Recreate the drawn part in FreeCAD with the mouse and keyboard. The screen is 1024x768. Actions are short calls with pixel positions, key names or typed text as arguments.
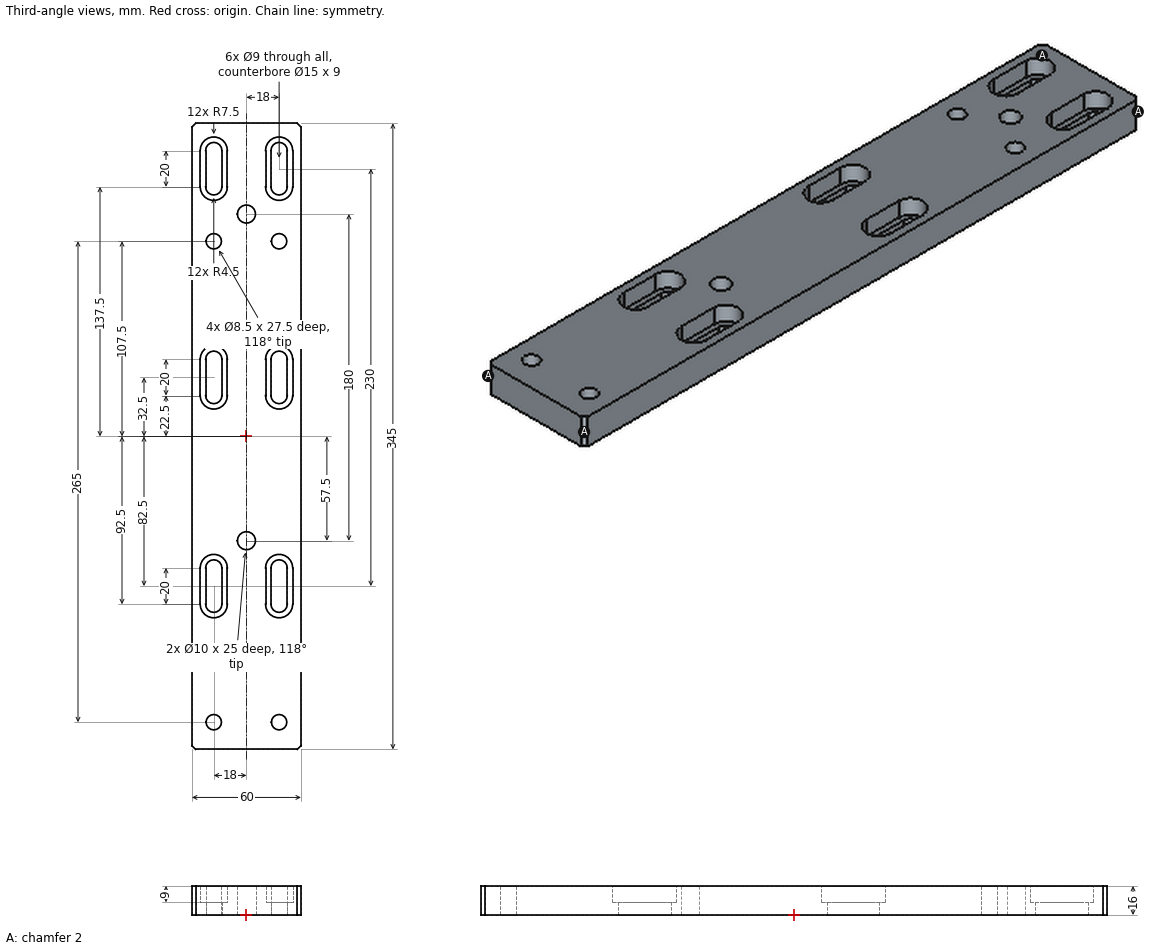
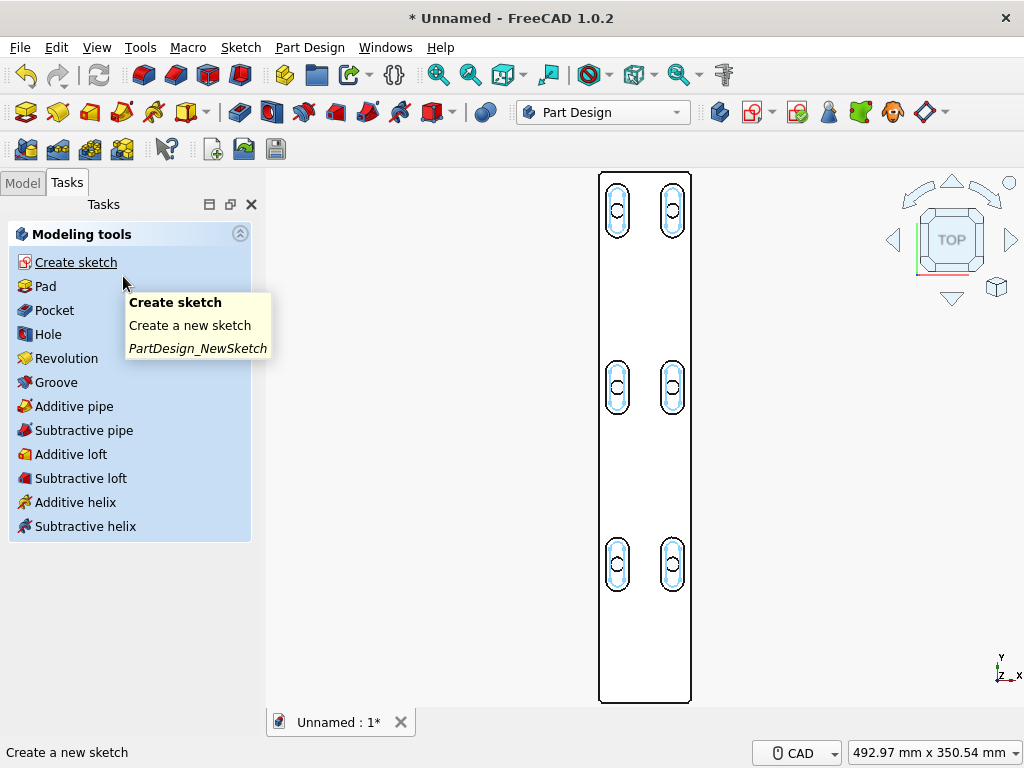
click(240, 112)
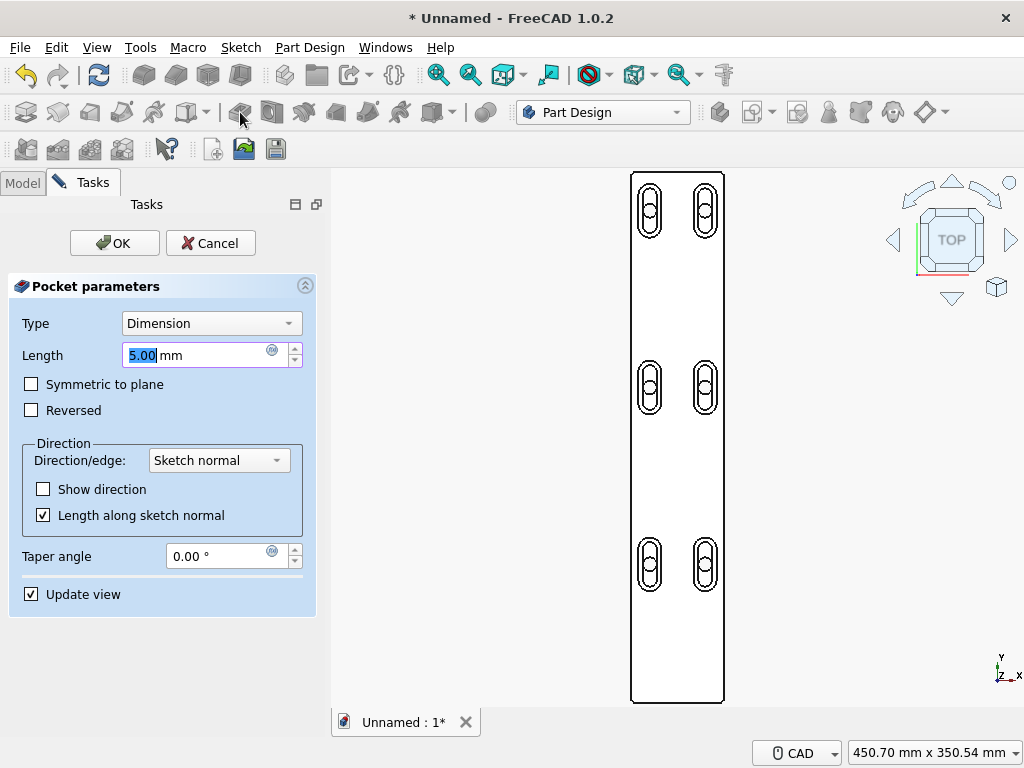
click(212, 324)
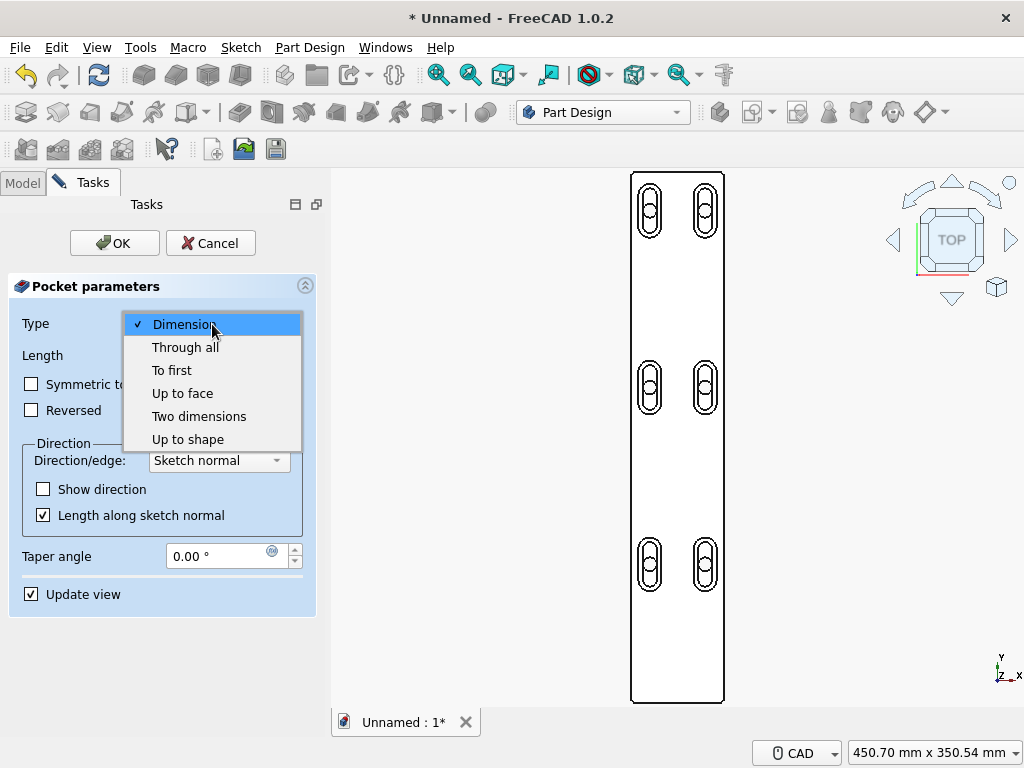
click(212, 348)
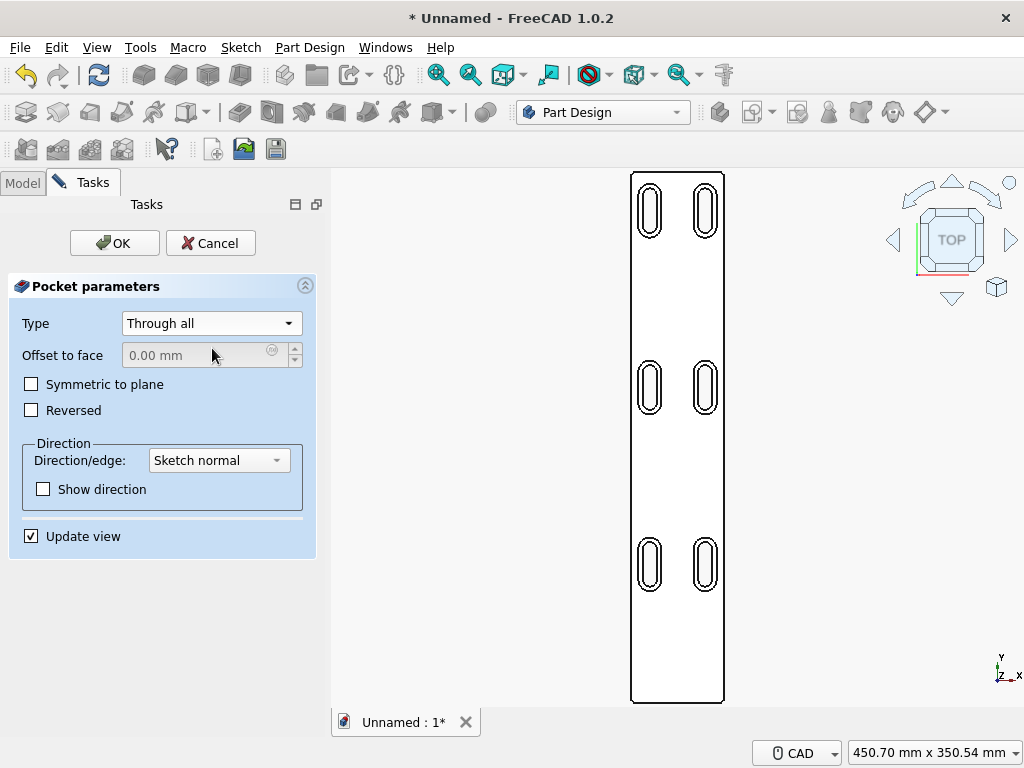
click(115, 243)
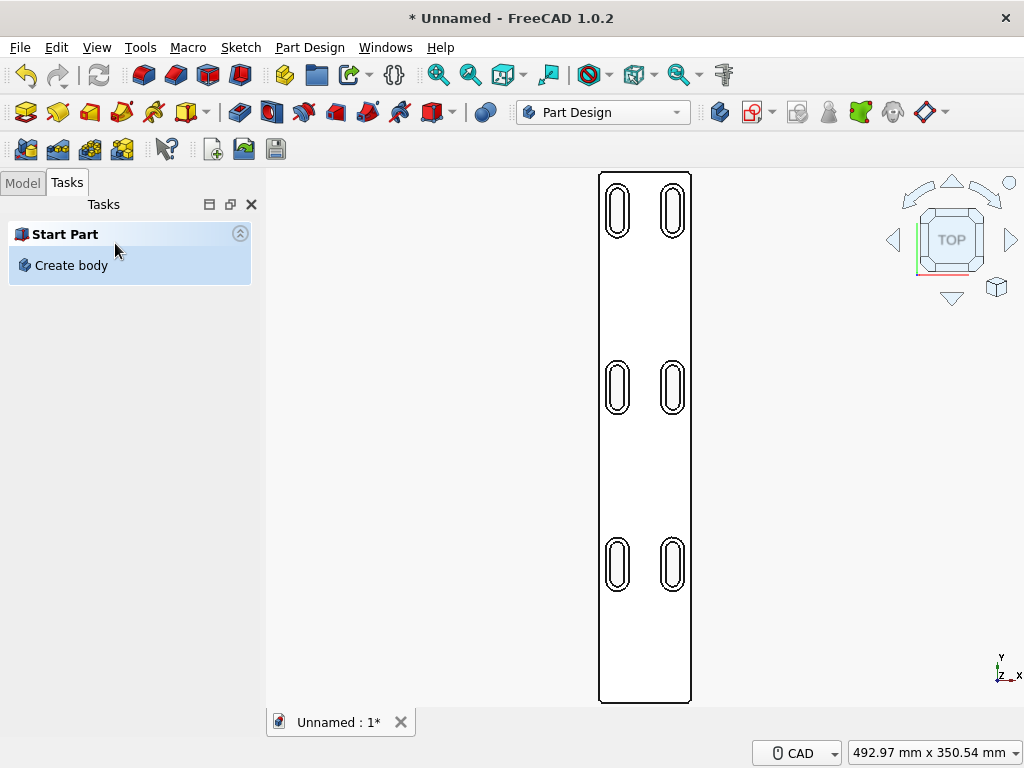
click(645, 285)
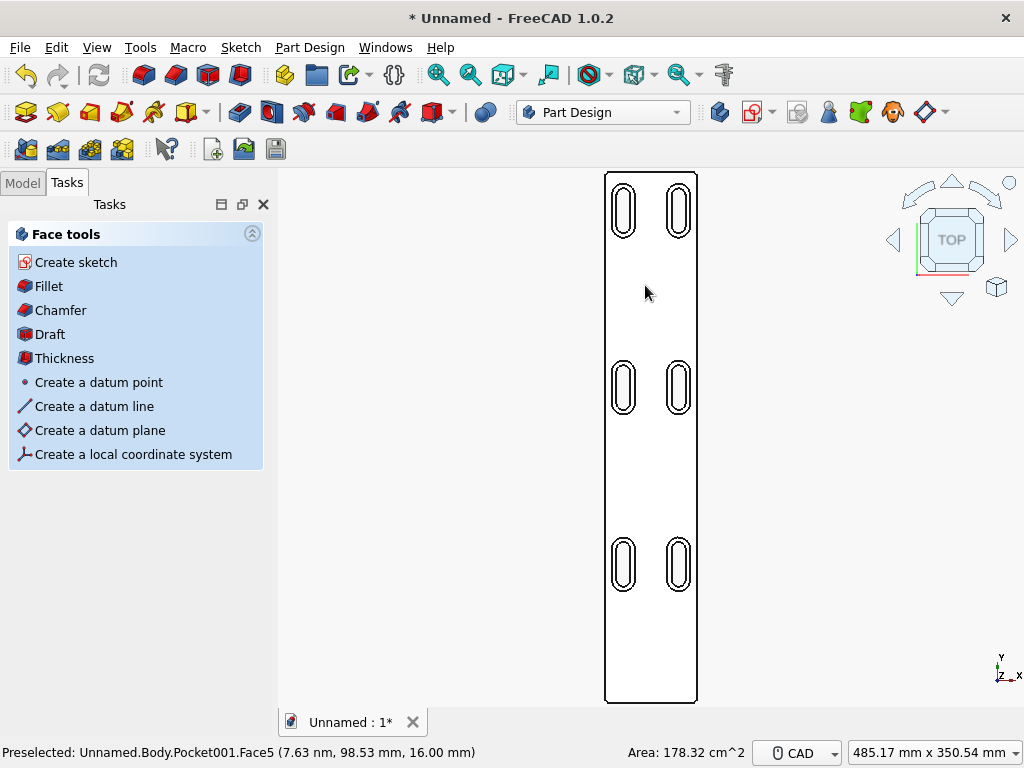
click(752, 112)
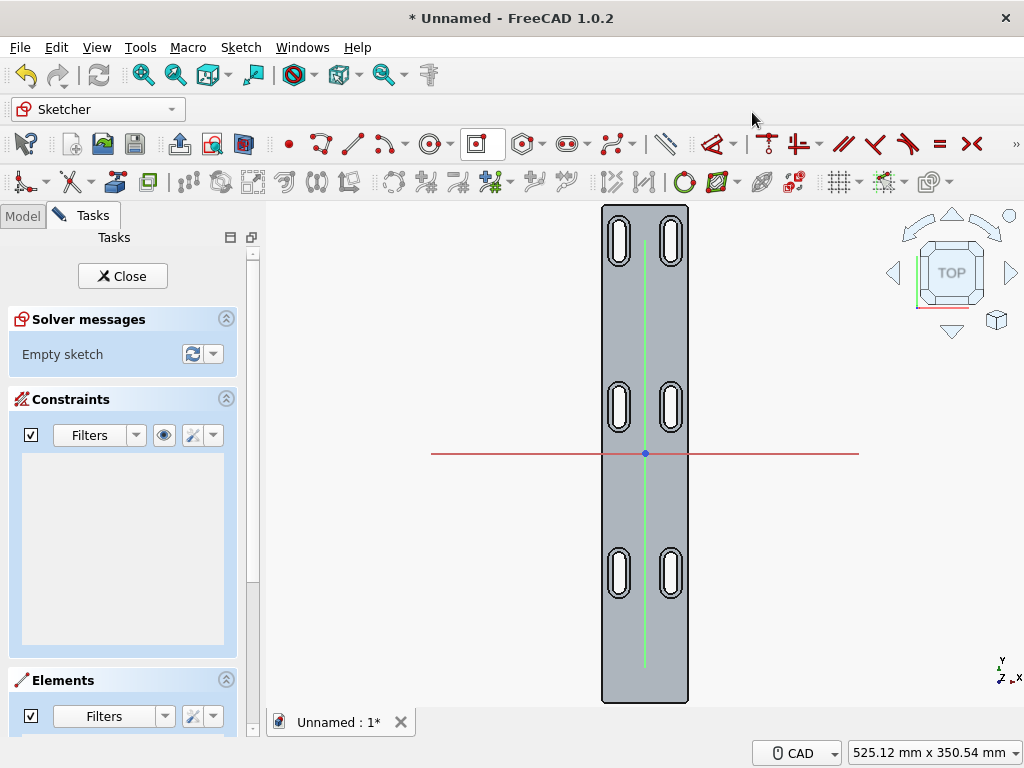
scroll(294, 291, down, 1)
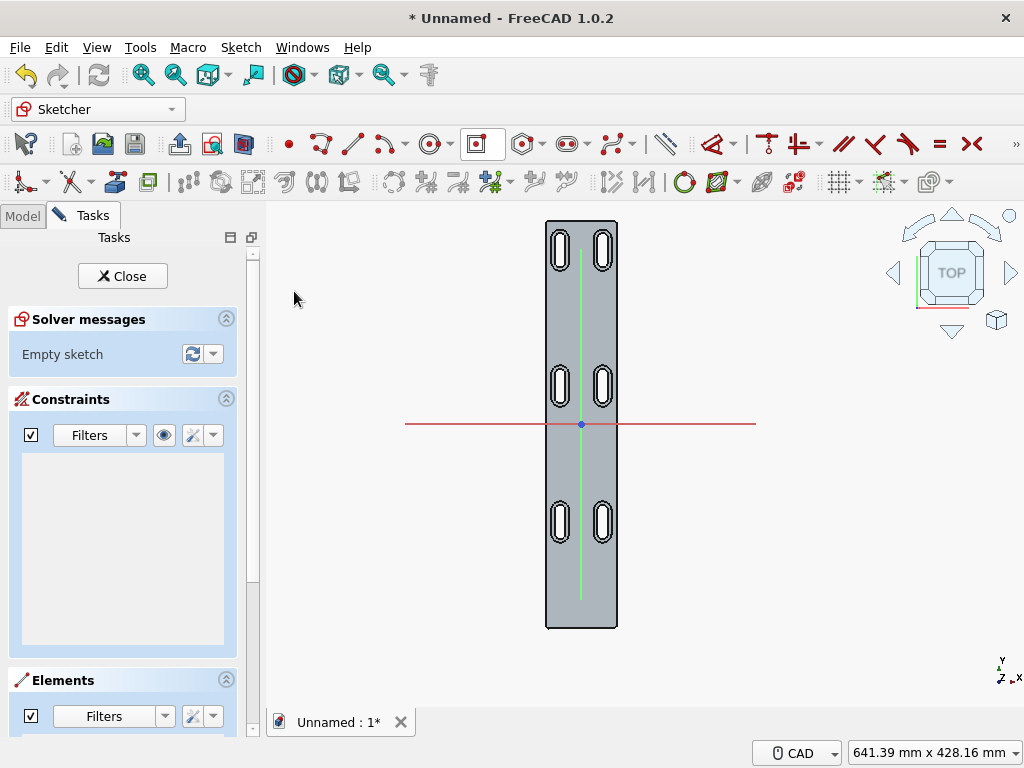
key(g)
key(c)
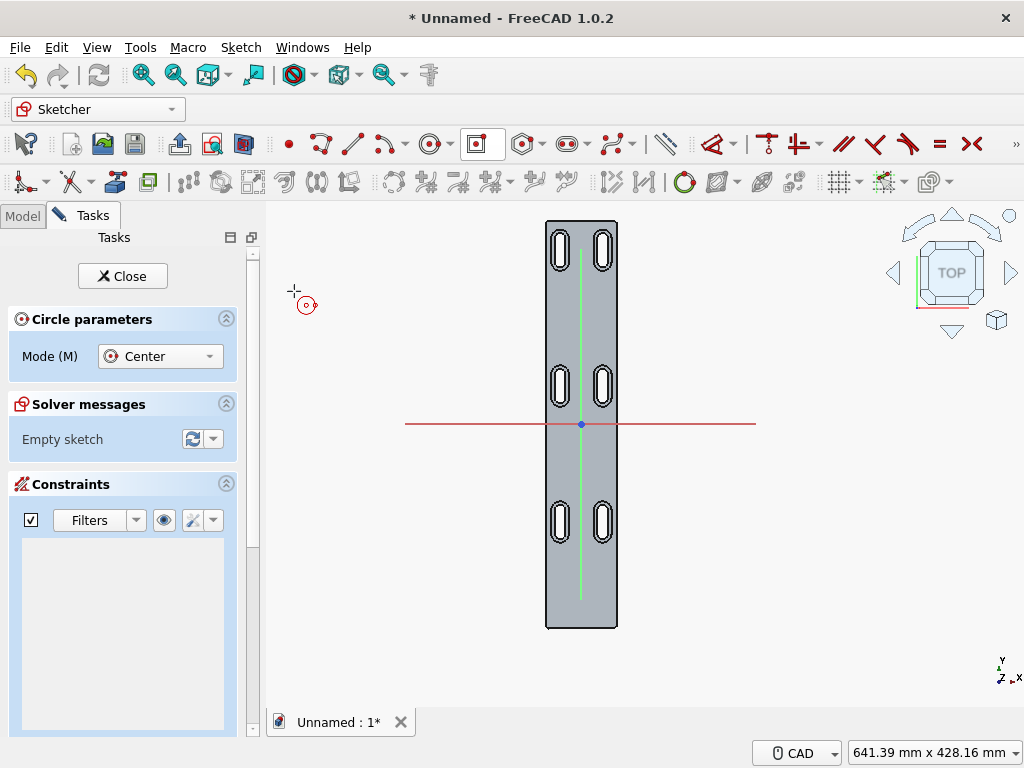
scroll(560, 297, up, 8)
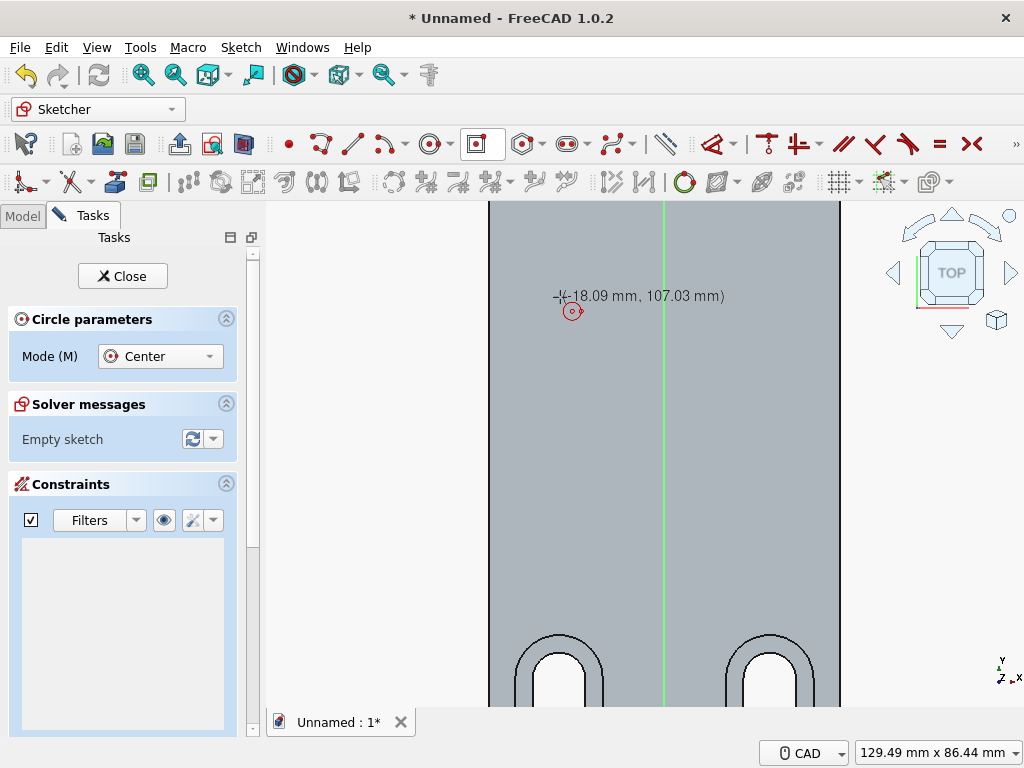
scroll(554, 297, down, 8)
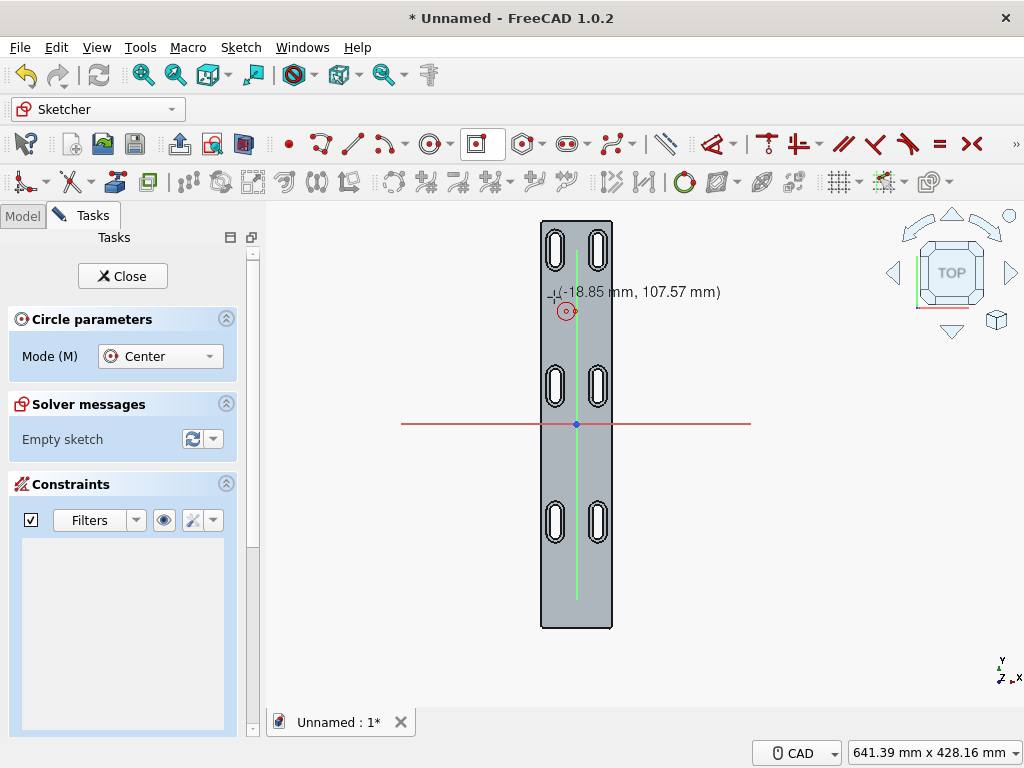
click(555, 297)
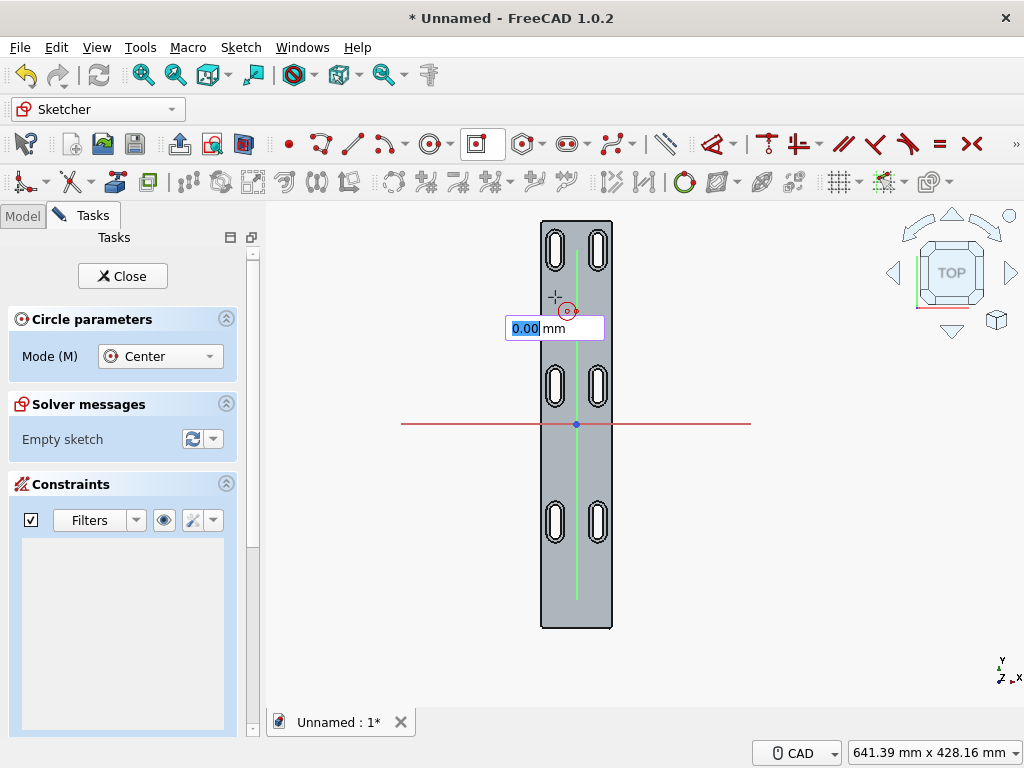
scroll(559, 294, up, 6)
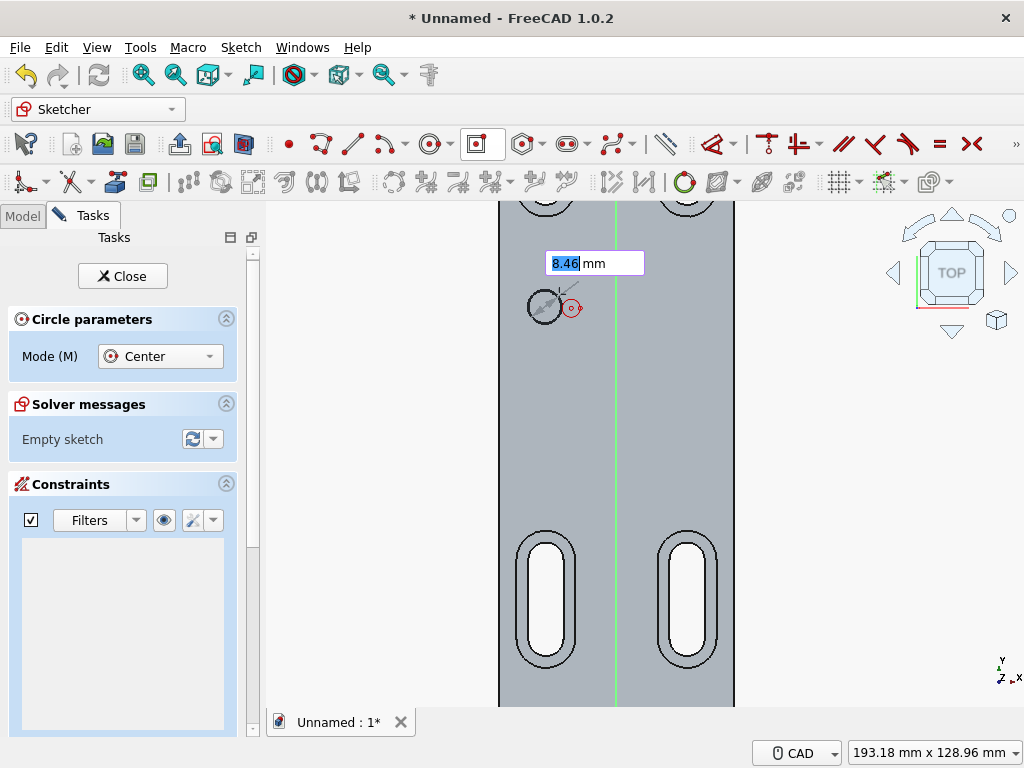
click(558, 293)